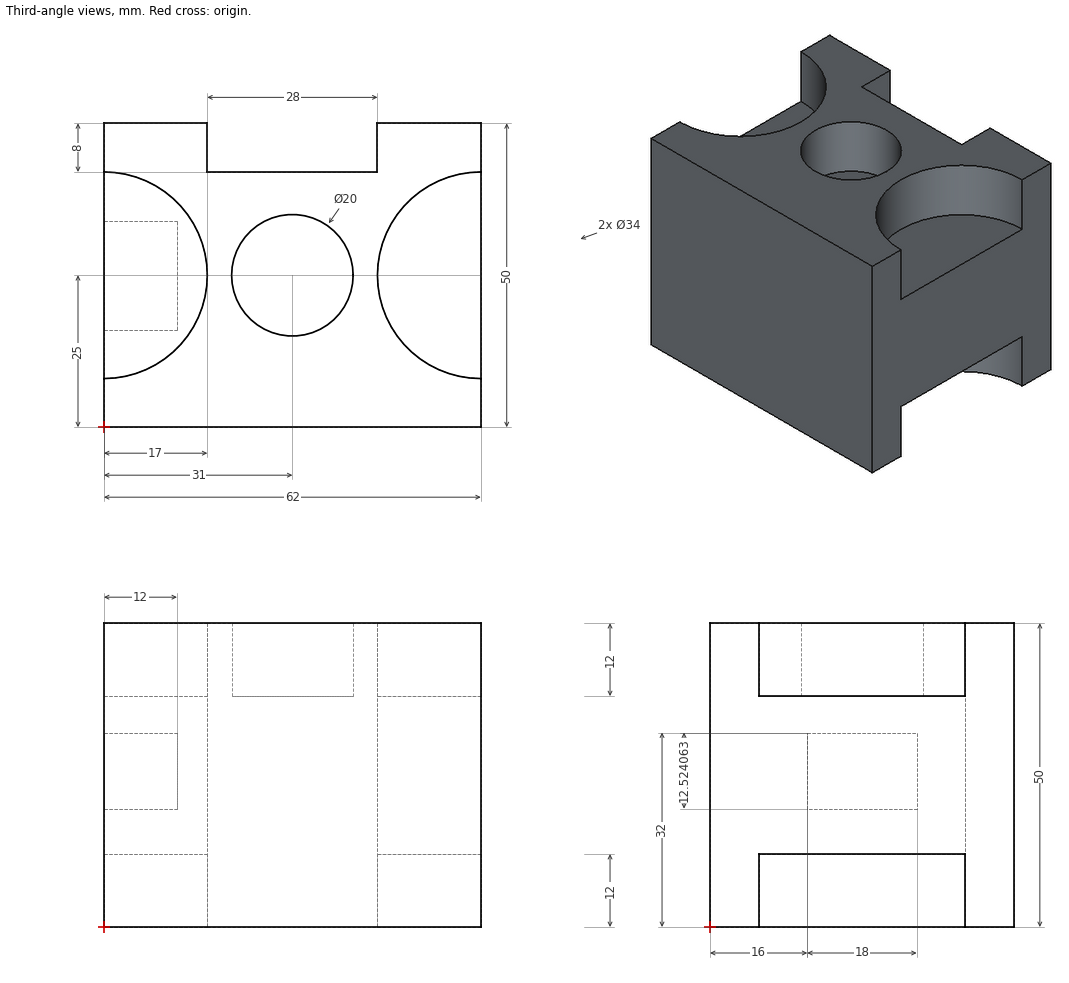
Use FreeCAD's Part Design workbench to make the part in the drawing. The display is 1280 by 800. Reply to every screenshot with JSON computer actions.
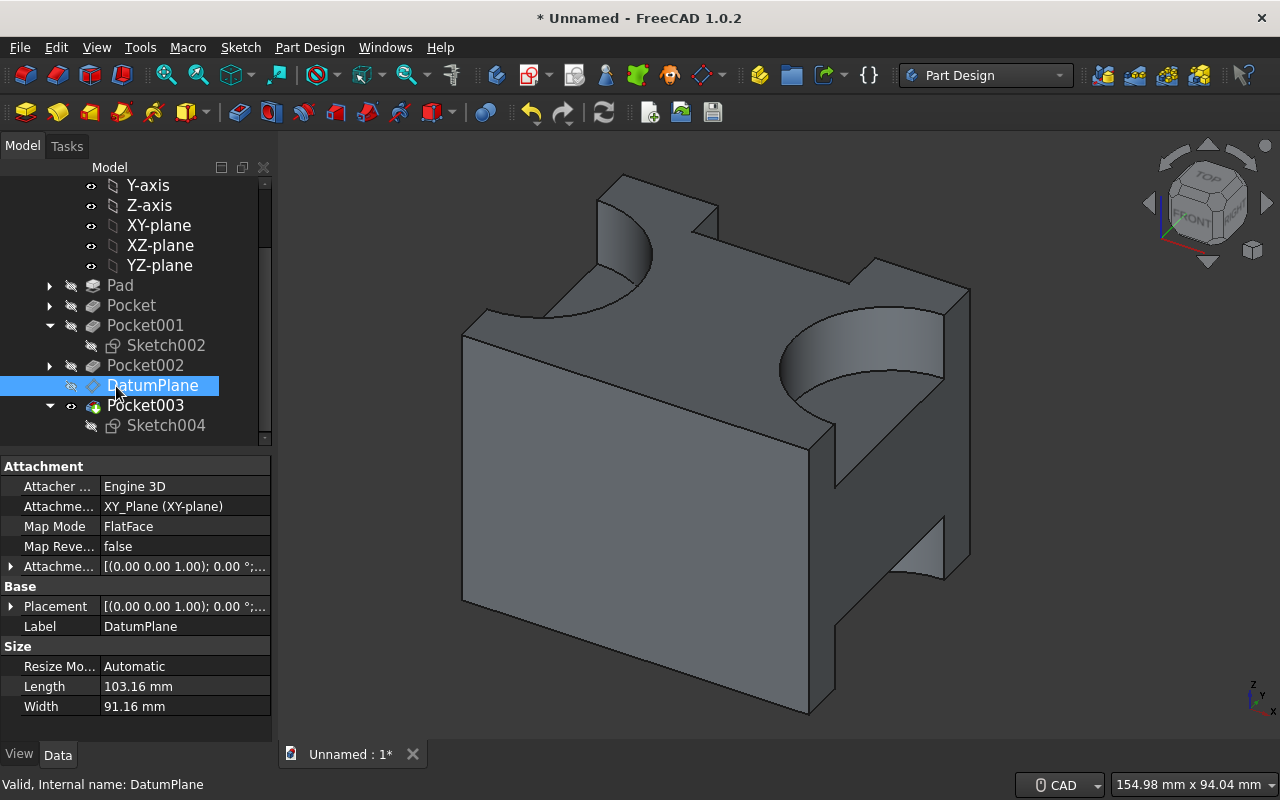
{"action": "left_click", "coordinate": [693, 334]}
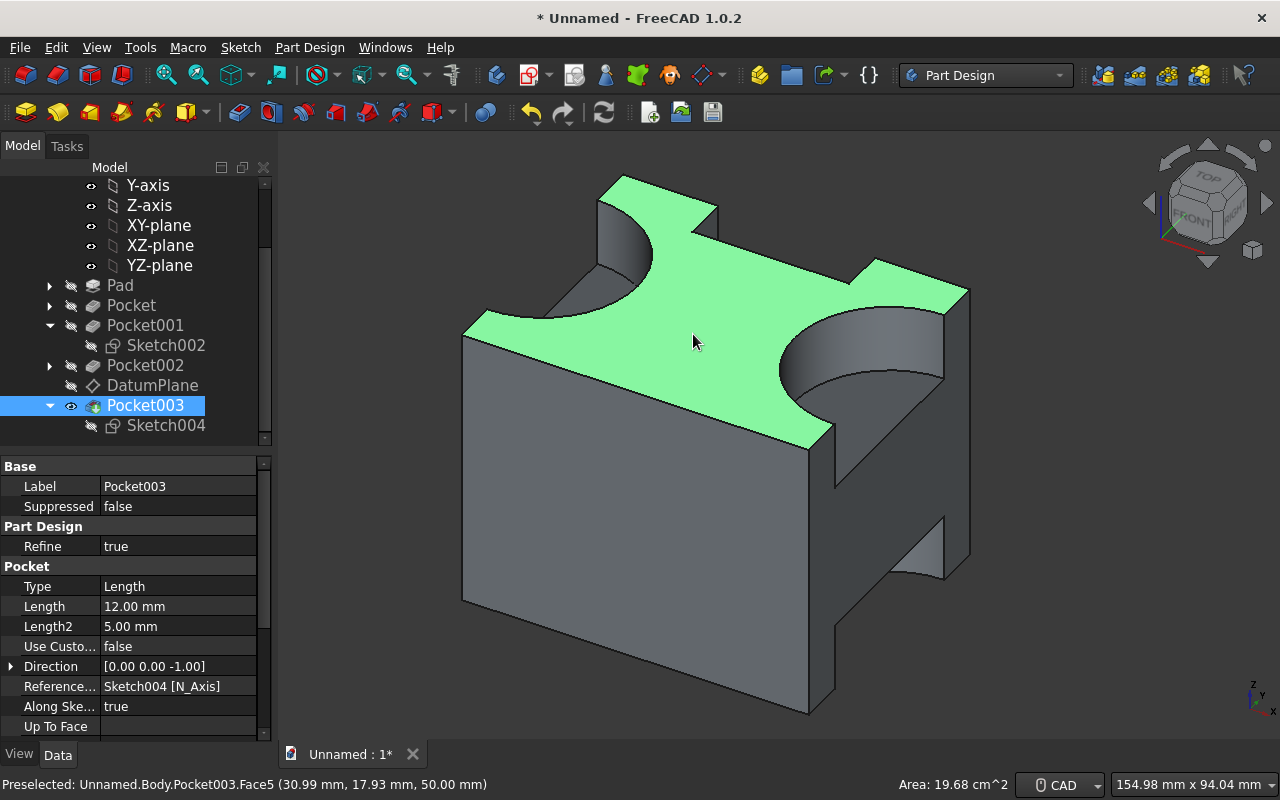
{"action": "left_click", "coordinate": [530, 76]}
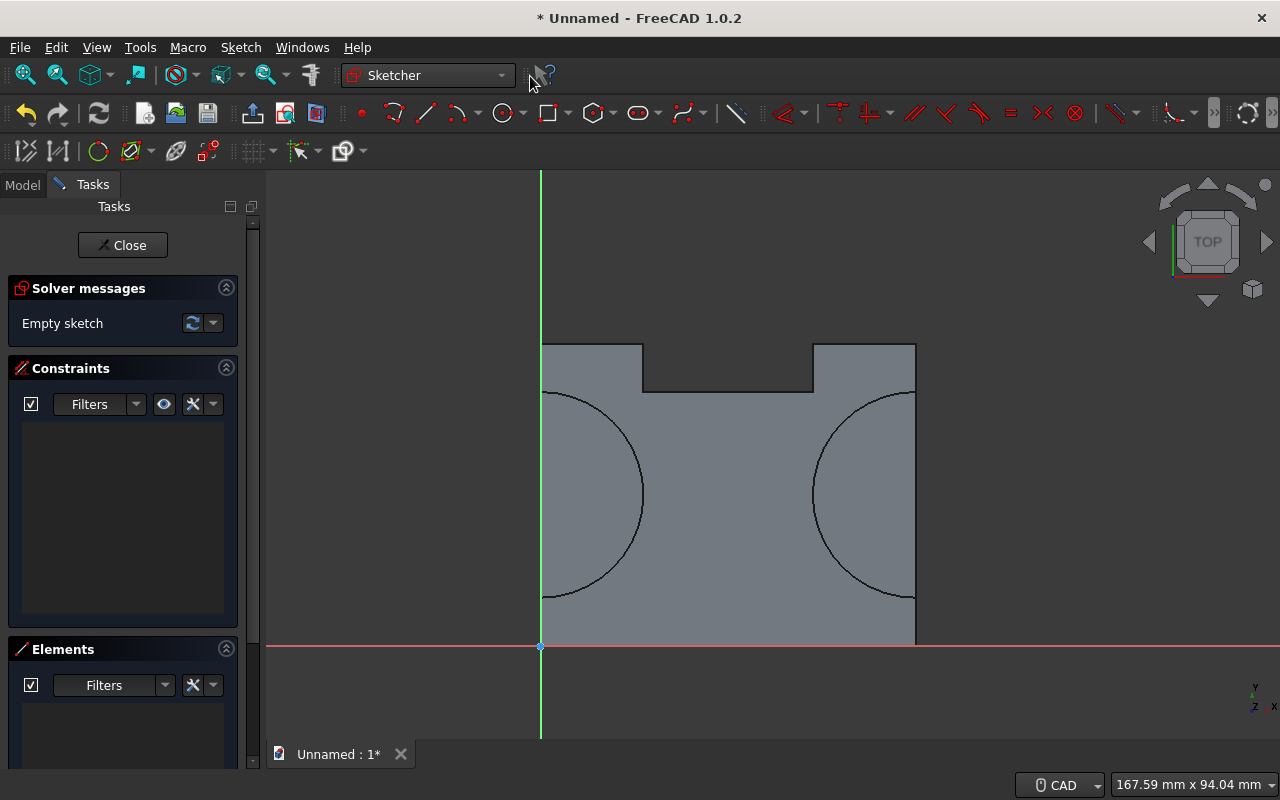
{"action": "scroll", "coordinate": [616, 645], "scroll_direction": "up", "scroll_amount": 3}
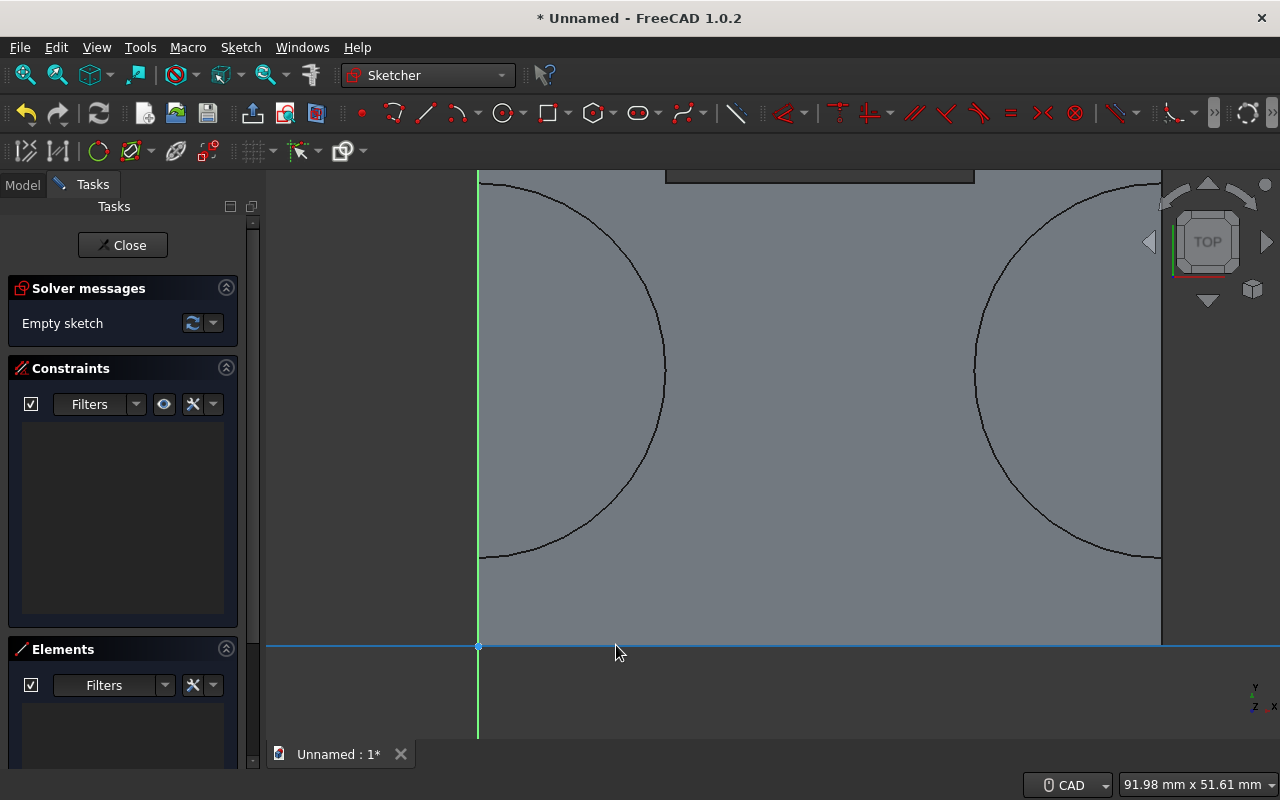
{"action": "left_click", "coordinate": [504, 114]}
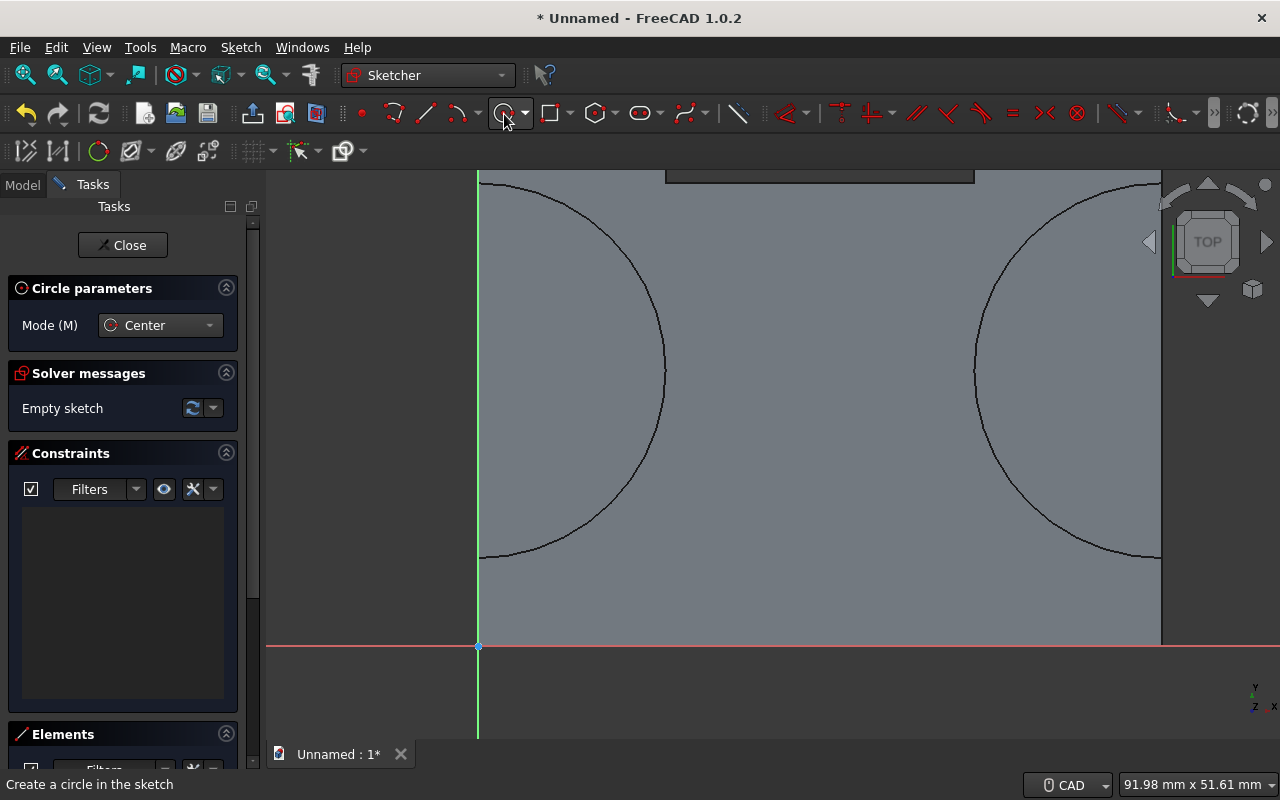
{"action": "left_click", "coordinate": [820, 371]}
{"action": "left_click", "coordinate": [898, 293]}
{"action": "key", "text": "Escape"}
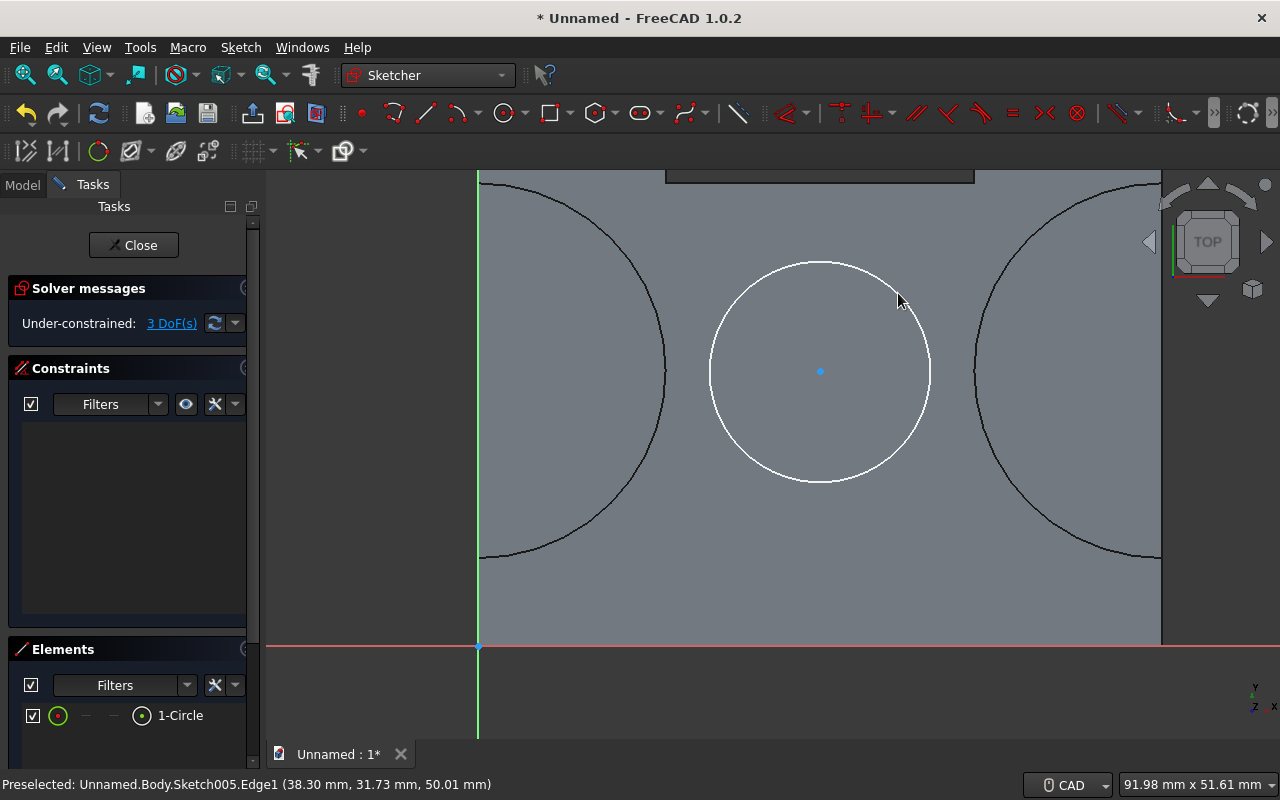
{"action": "left_click", "coordinate": [786, 114]}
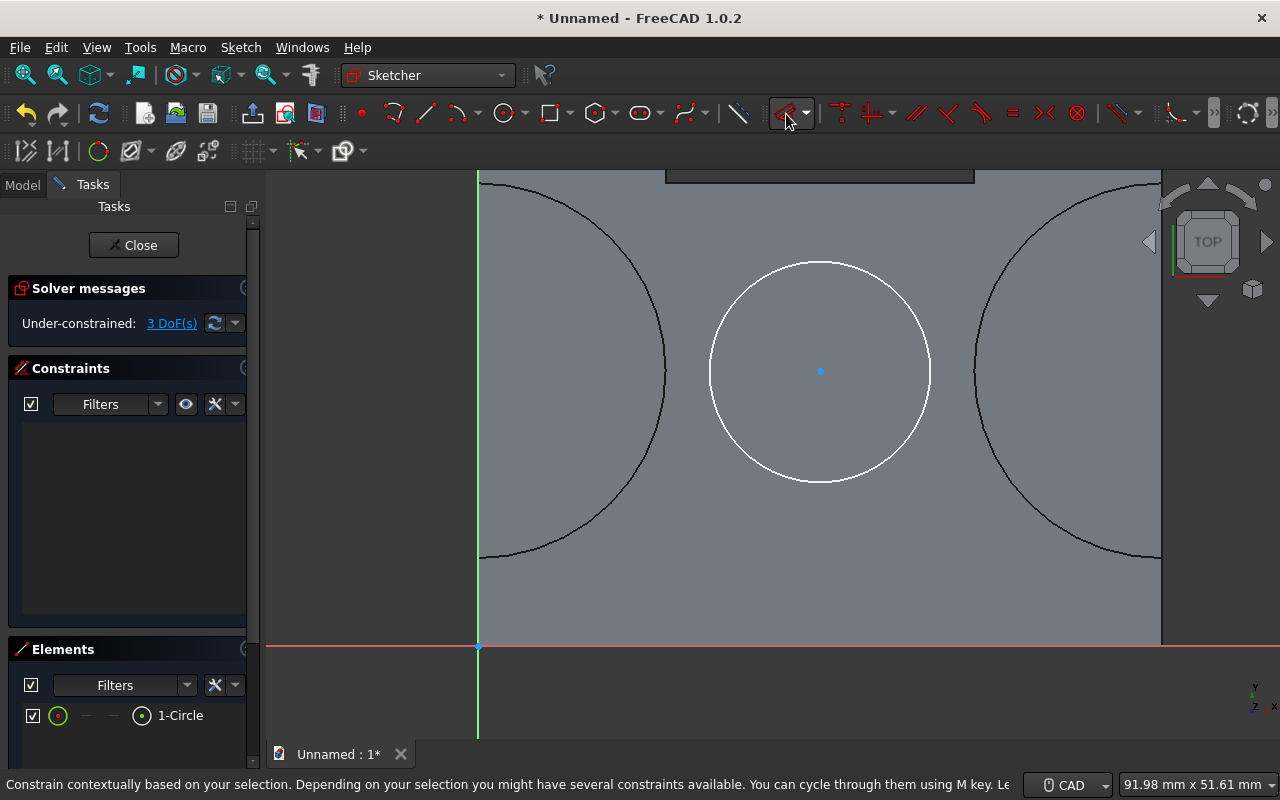
{"action": "left_click", "coordinate": [898, 294]}
{"action": "left_click", "coordinate": [921, 271]}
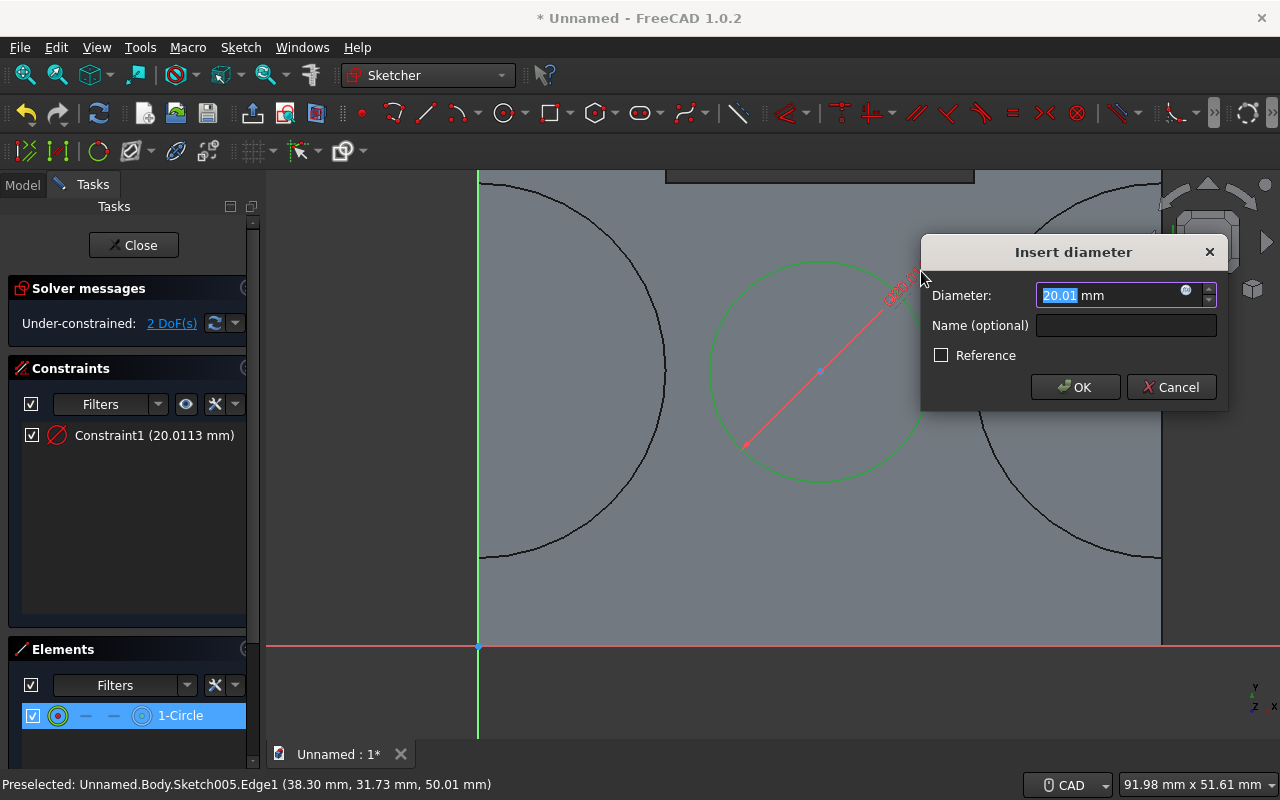
{"action": "type", "text": "20"}
{"action": "key", "text": "Return"}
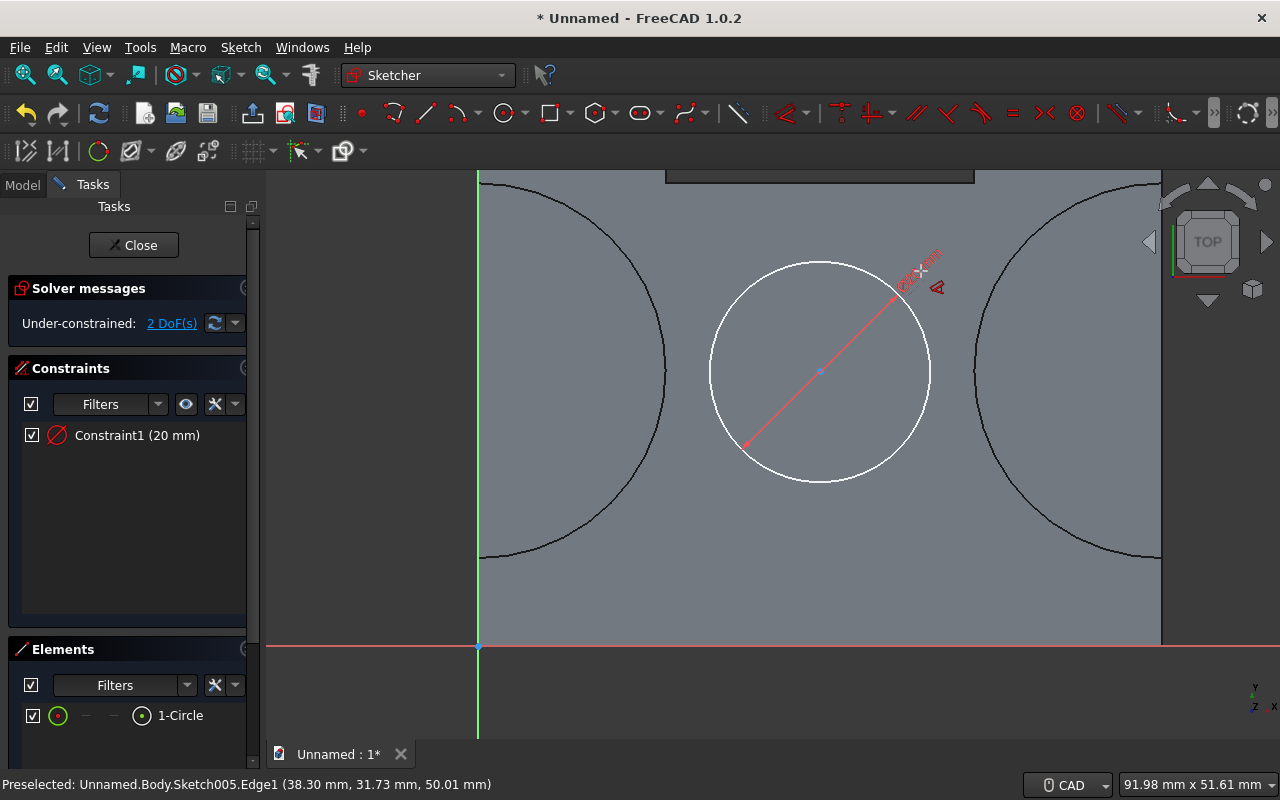
{"action": "left_click", "coordinate": [820, 372]}
{"action": "left_click", "coordinate": [649, 680]}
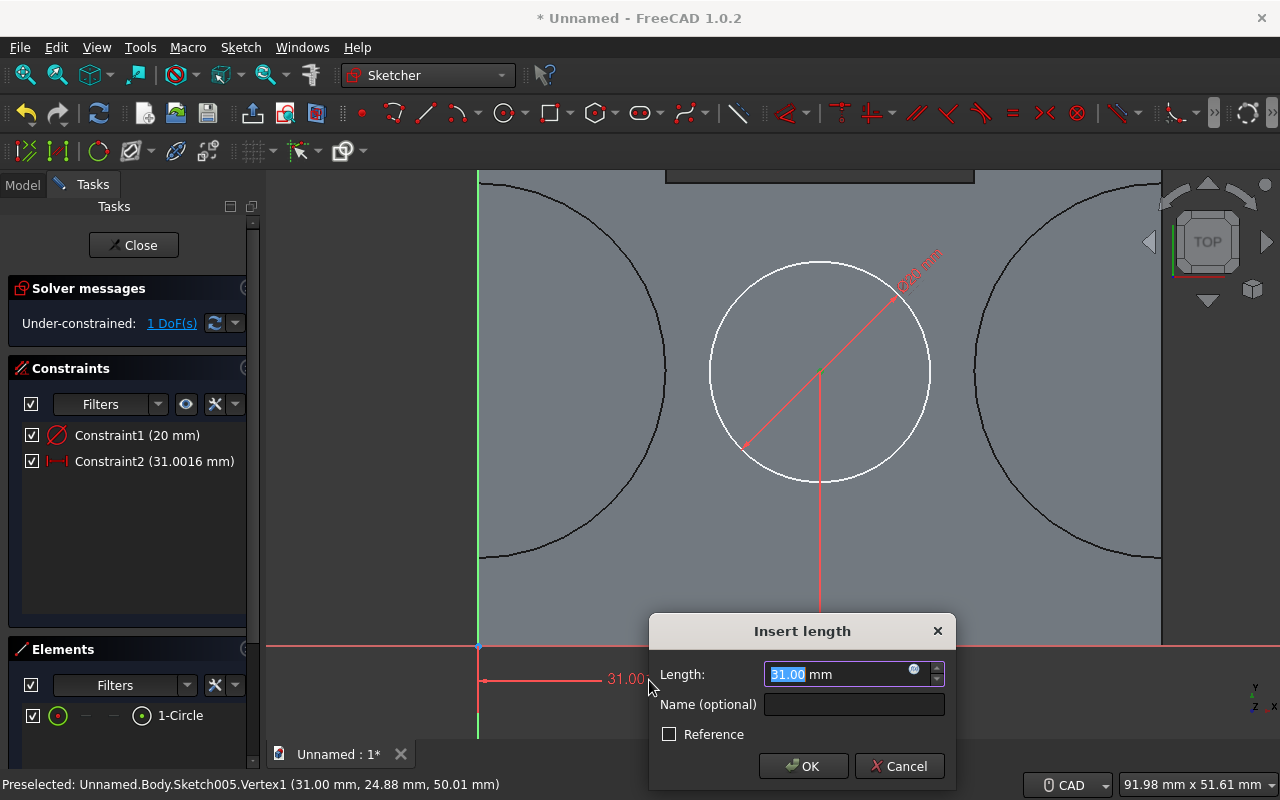
{"action": "type", "text": "31"}
{"action": "key", "text": "Return"}